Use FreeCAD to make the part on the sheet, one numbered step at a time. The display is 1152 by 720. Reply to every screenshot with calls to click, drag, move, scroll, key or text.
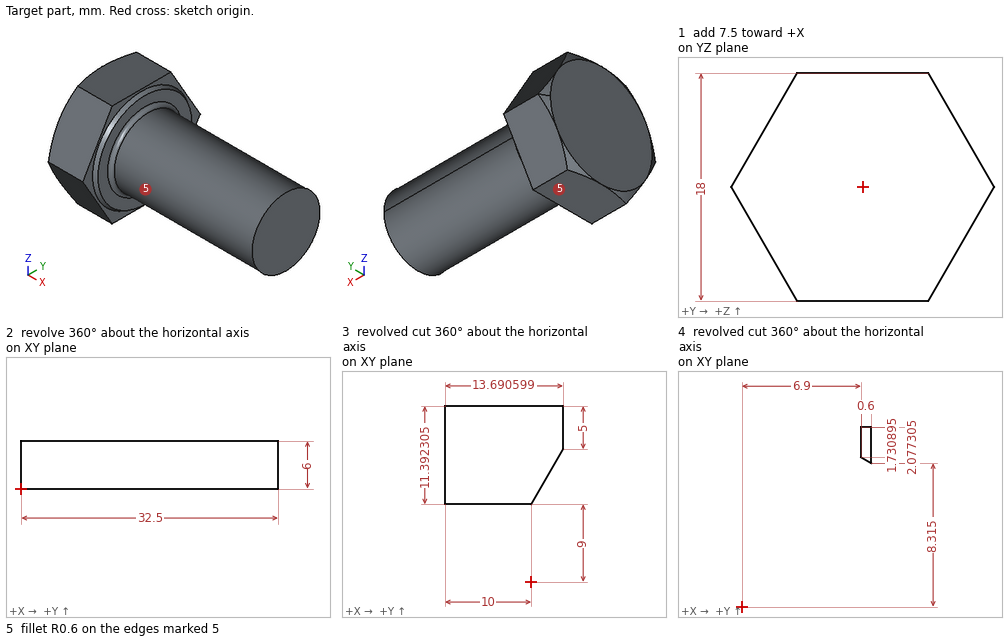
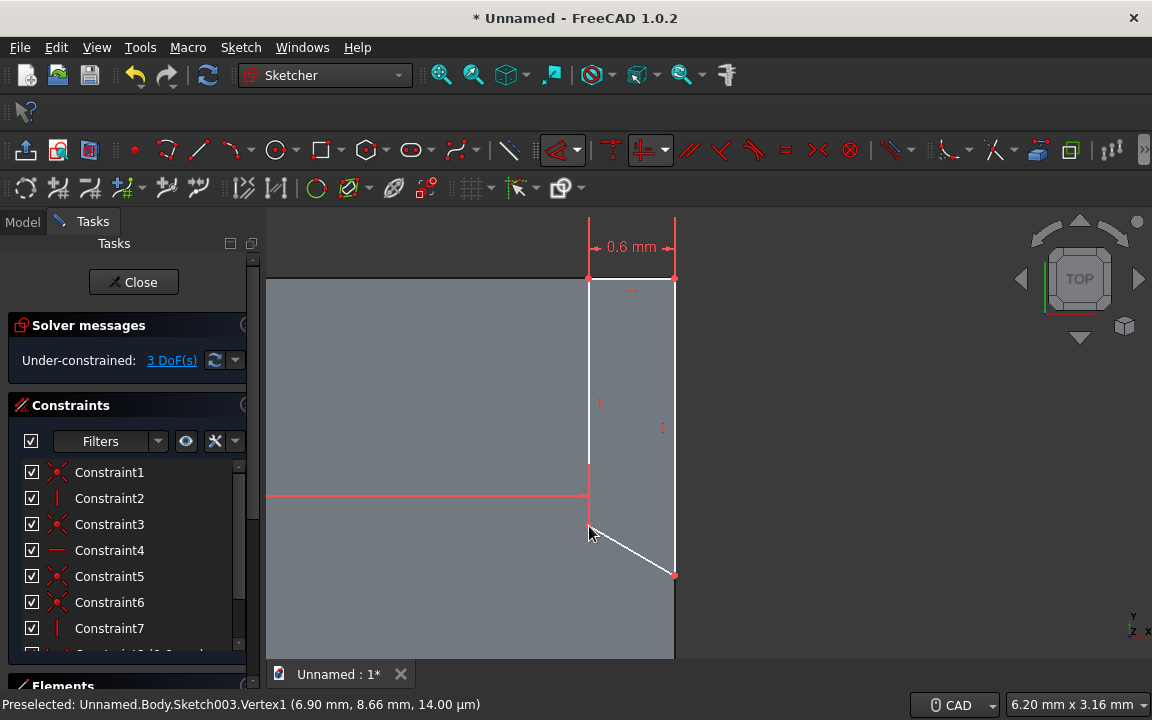
click(675, 576)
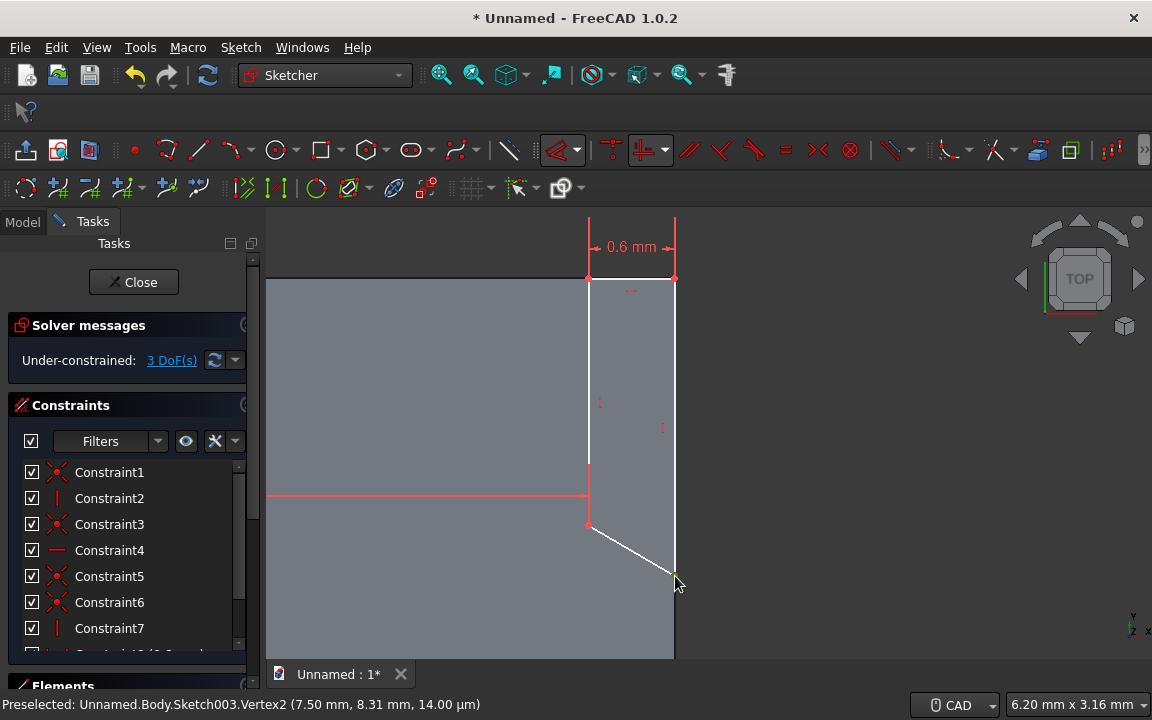
key(i)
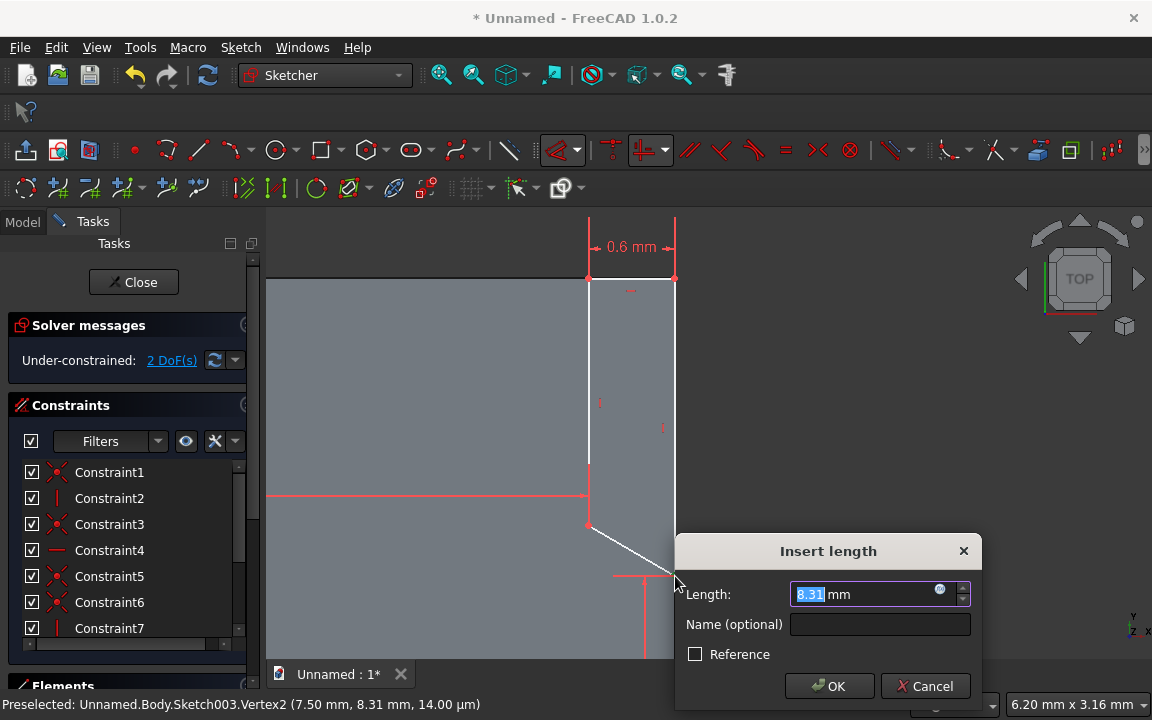
text(8.315)
key(Return)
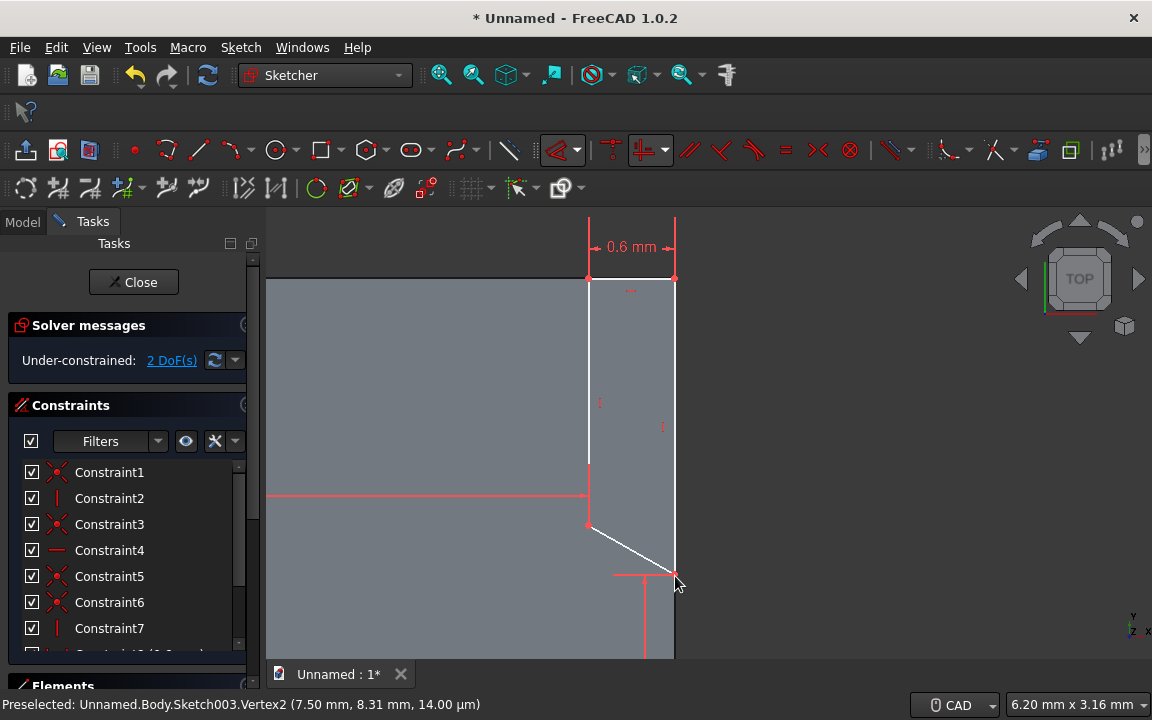
click(675, 486)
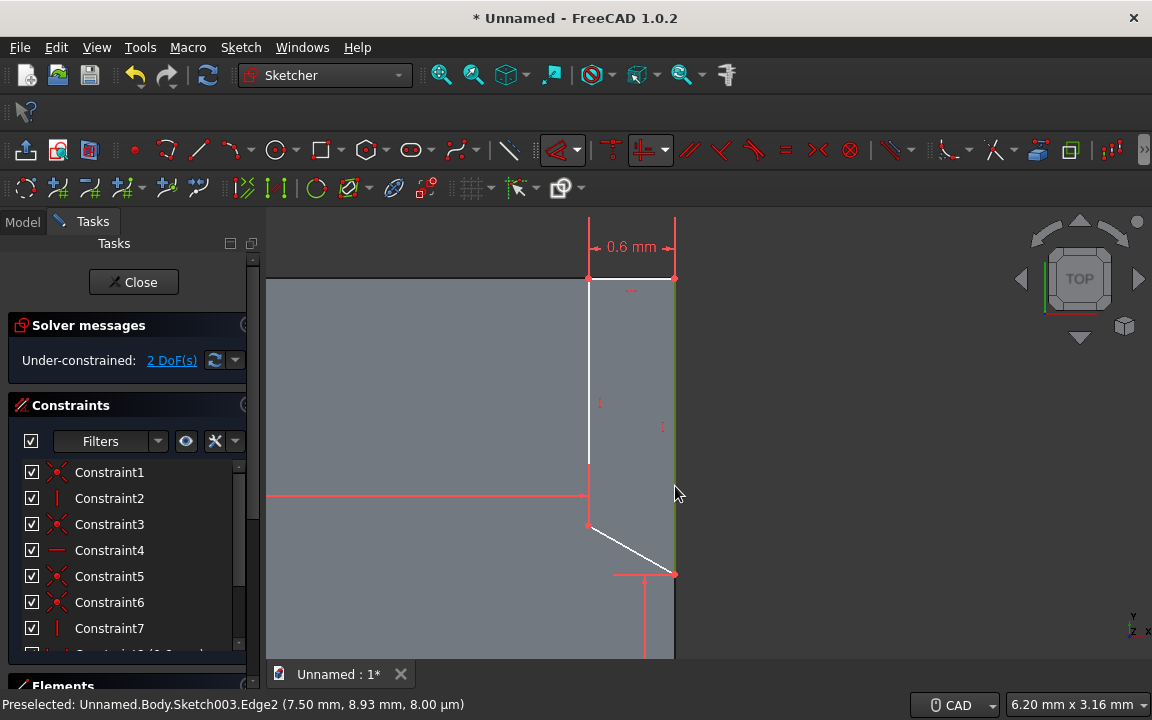
key(i)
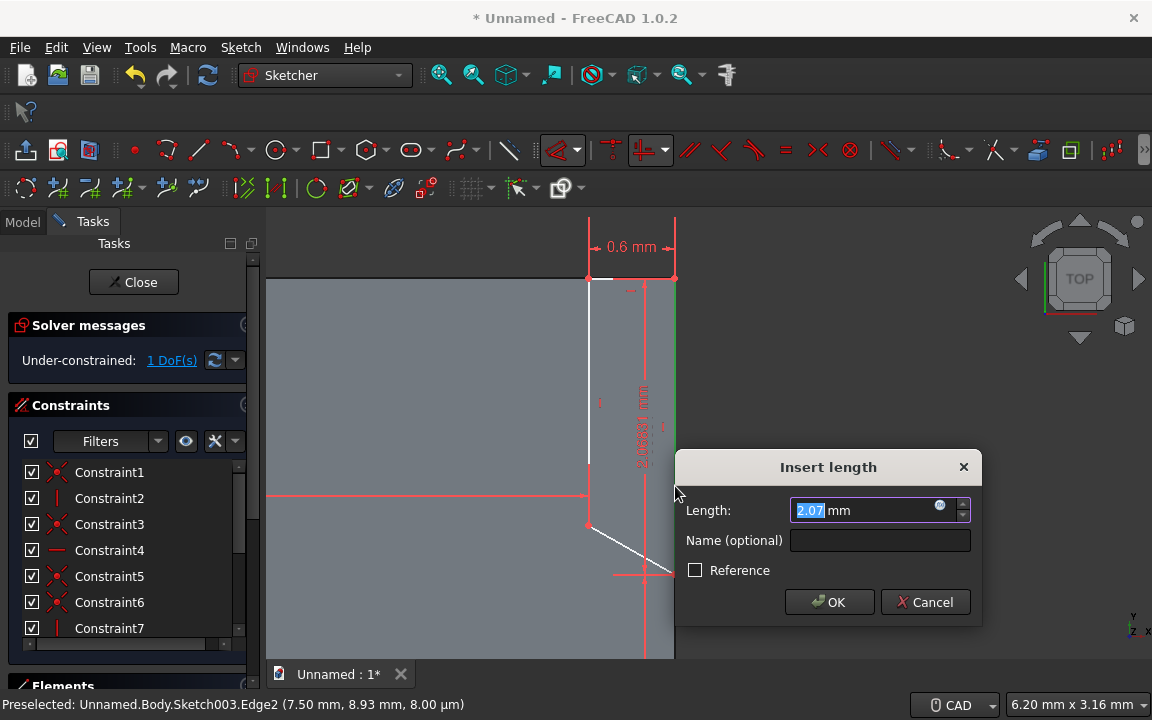
text(2.077305)
key(Return)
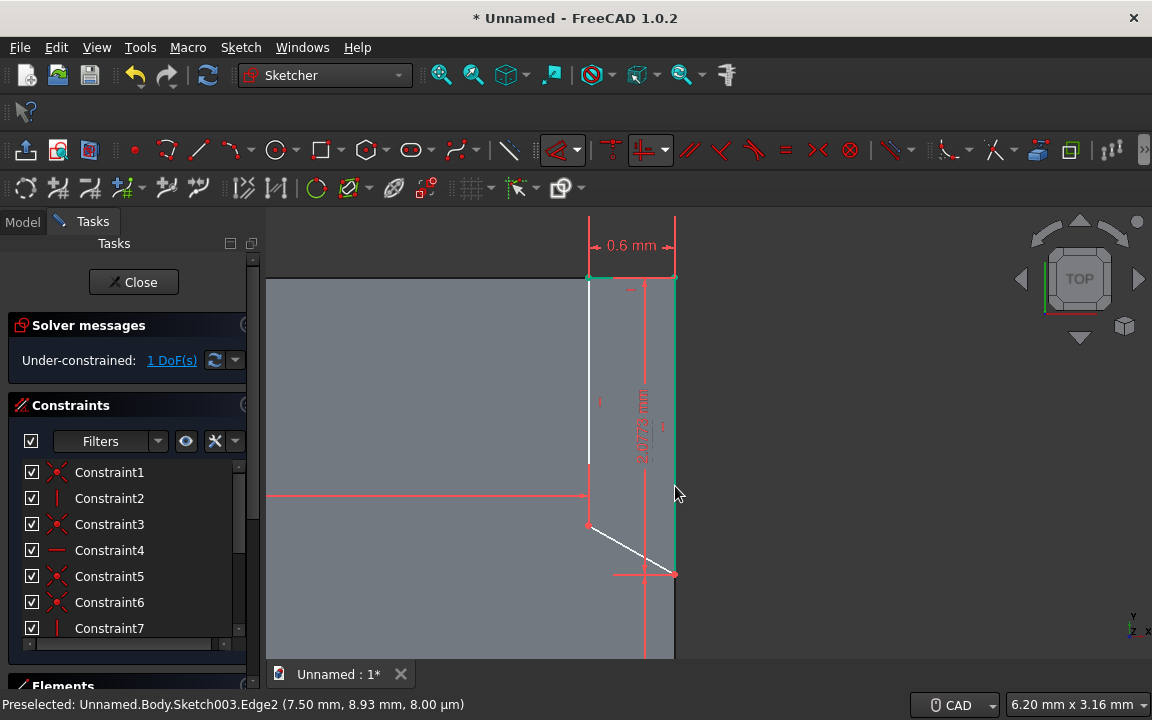
click(589, 352)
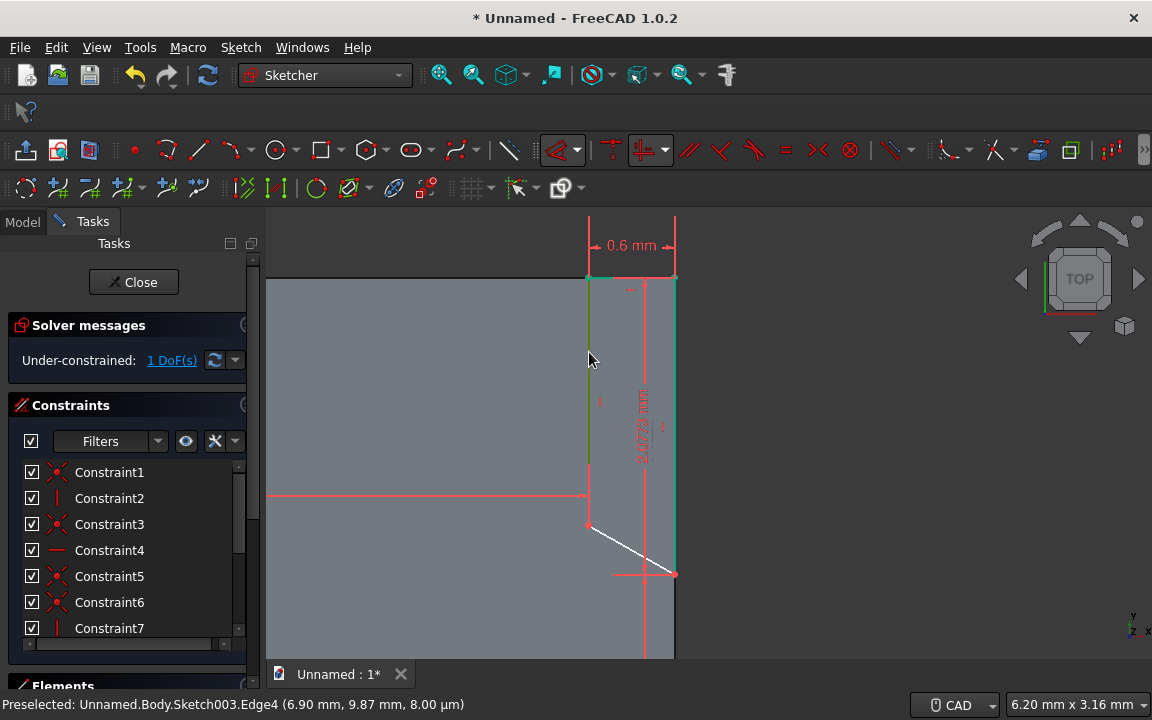
click(580, 150)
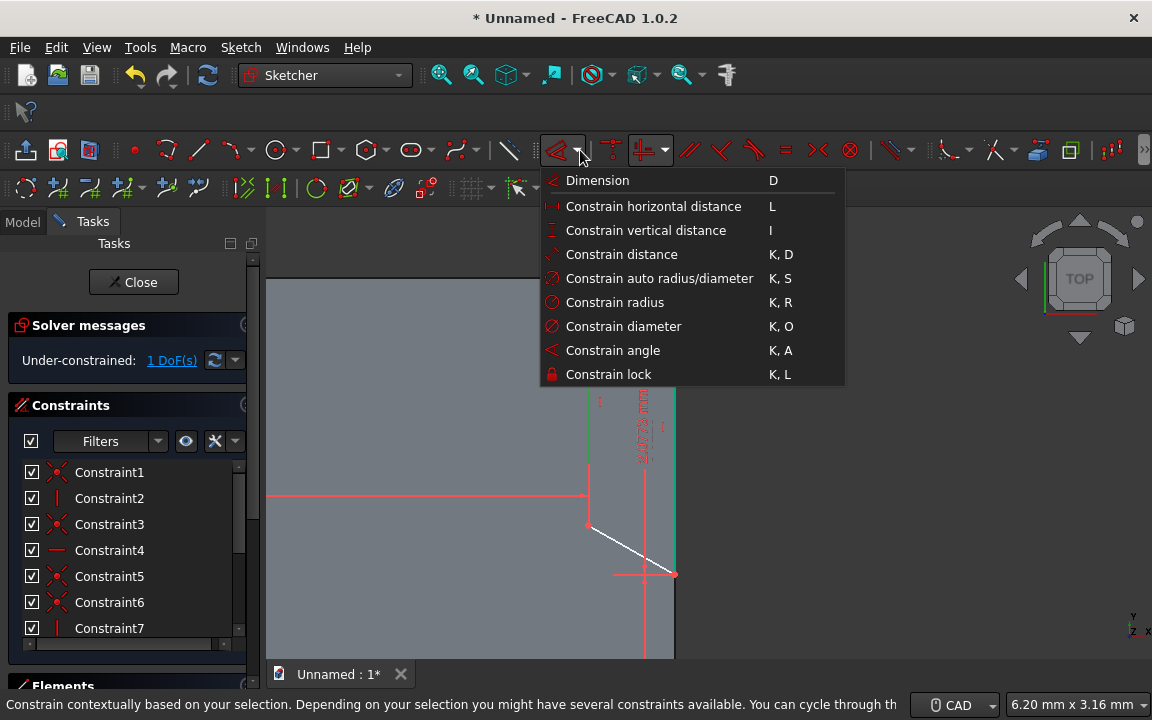
click(693, 230)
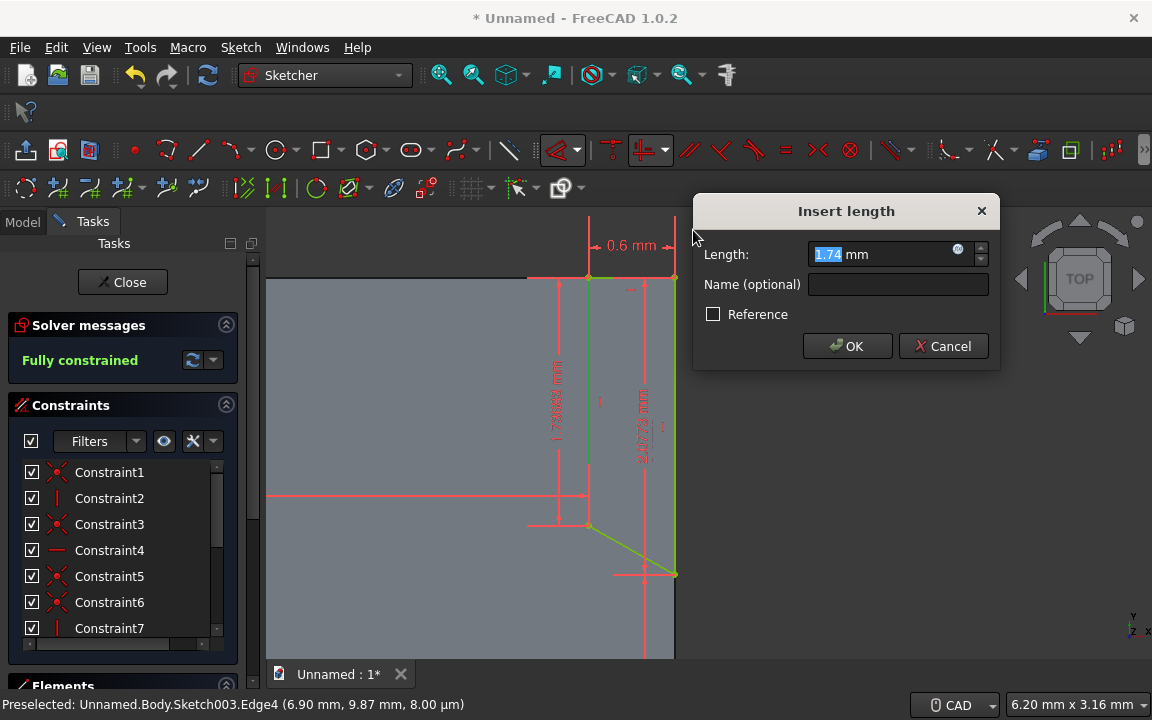
text(1.730895)
key(Return)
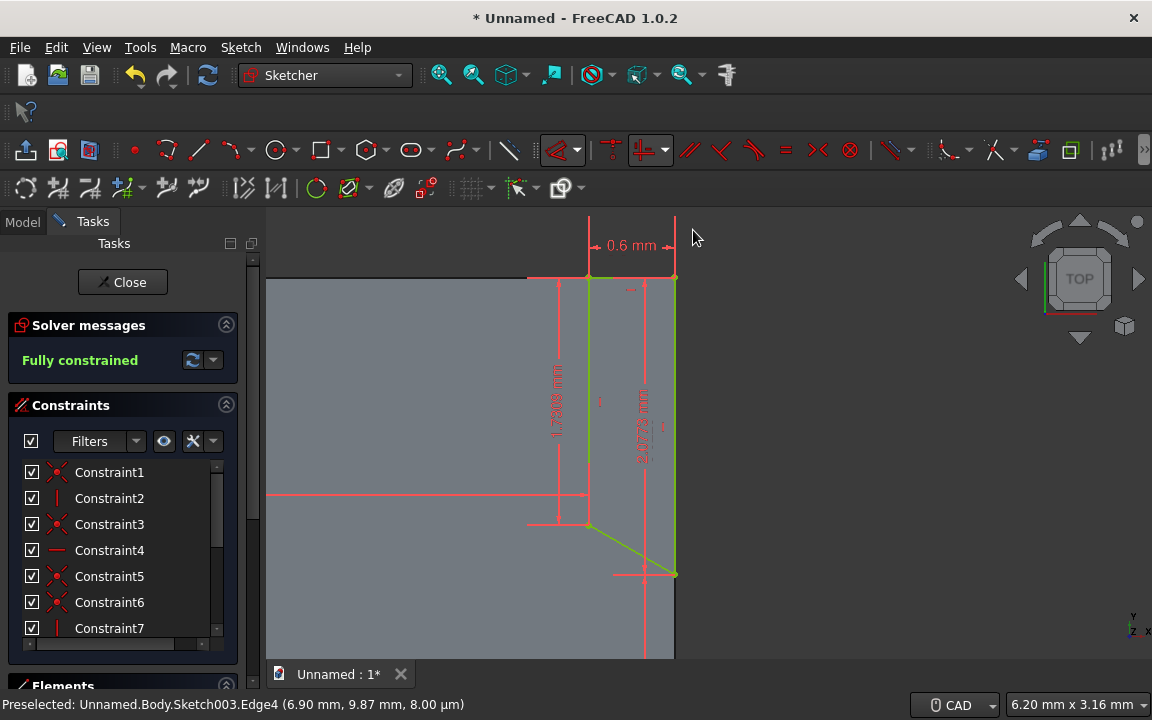
click(123, 282)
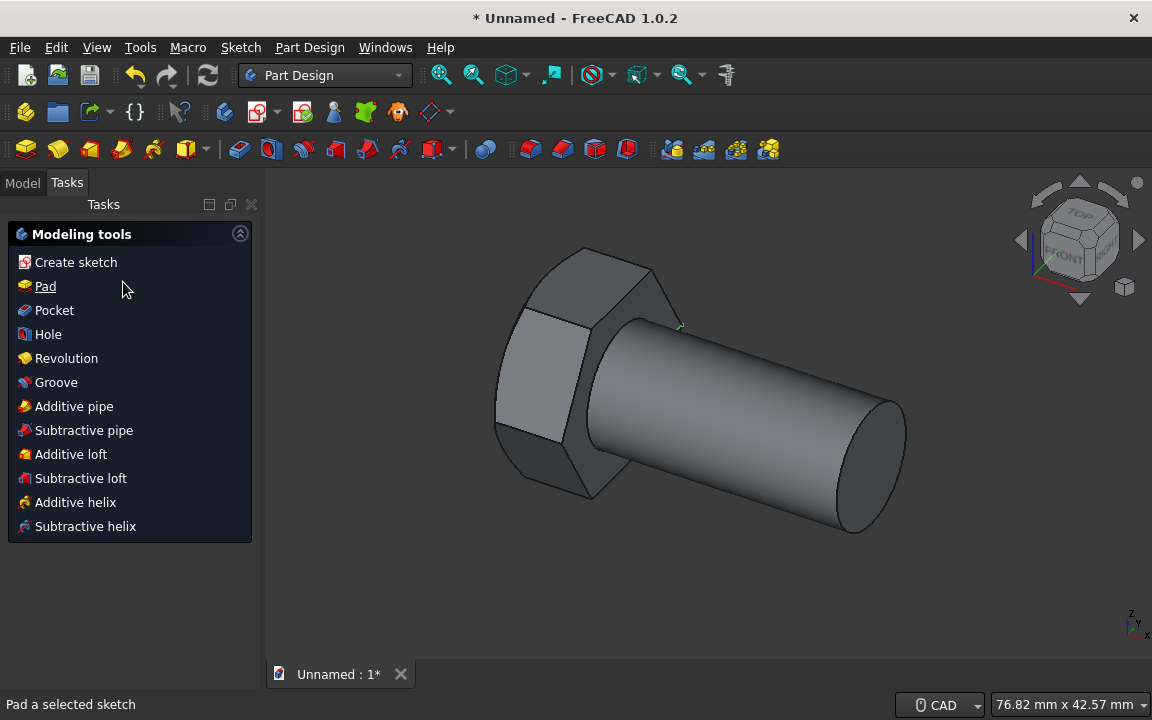
click(304, 150)